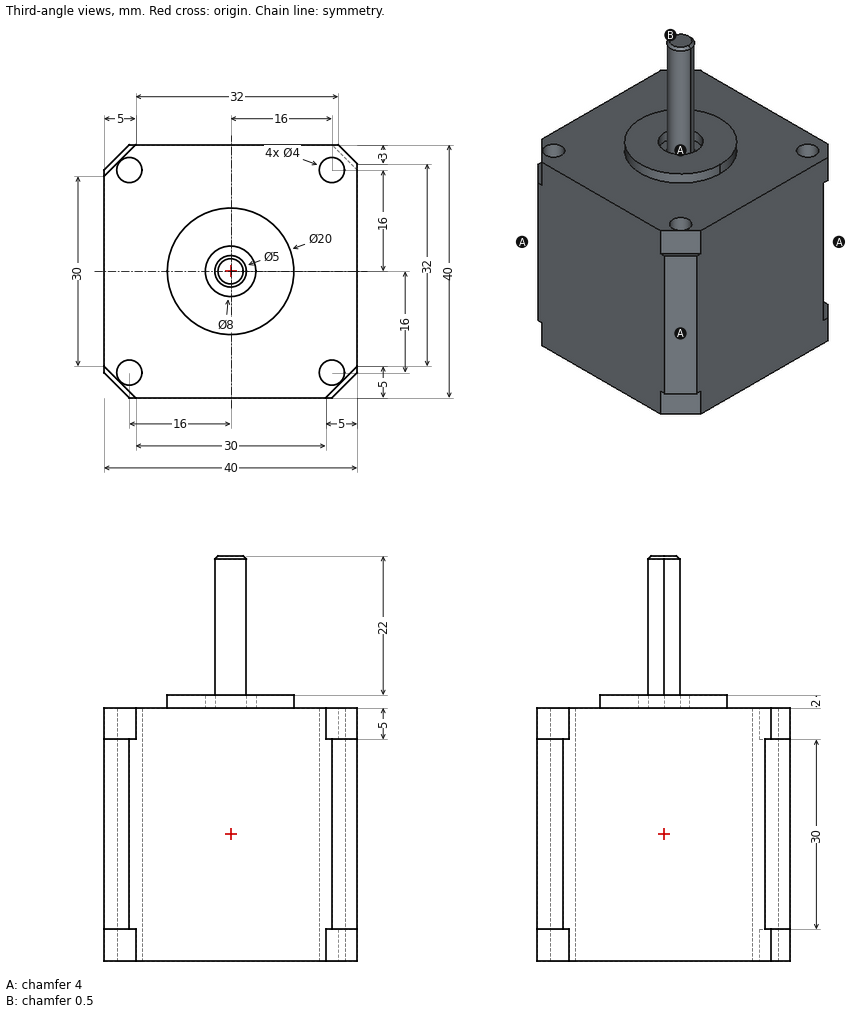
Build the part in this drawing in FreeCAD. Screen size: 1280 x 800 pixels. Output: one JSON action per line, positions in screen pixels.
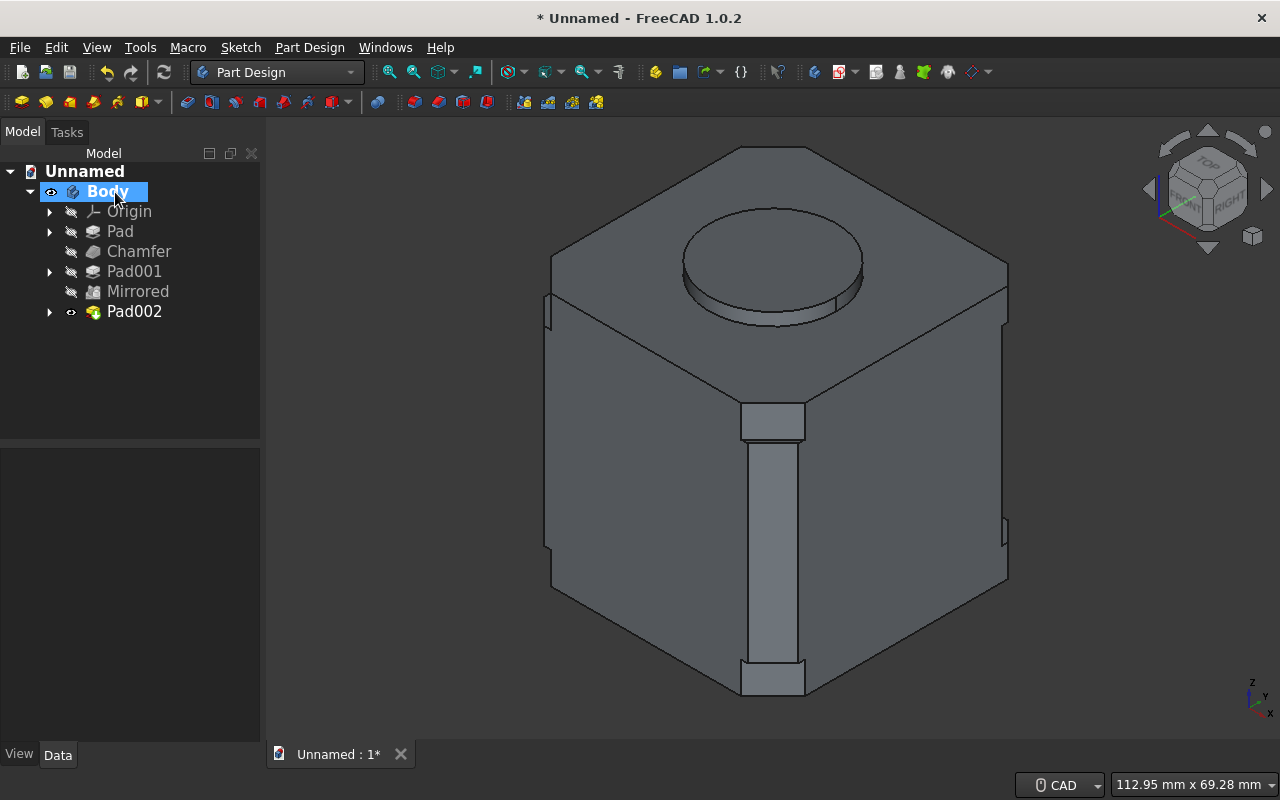
{"action": "left_click", "coordinate": [390, 72]}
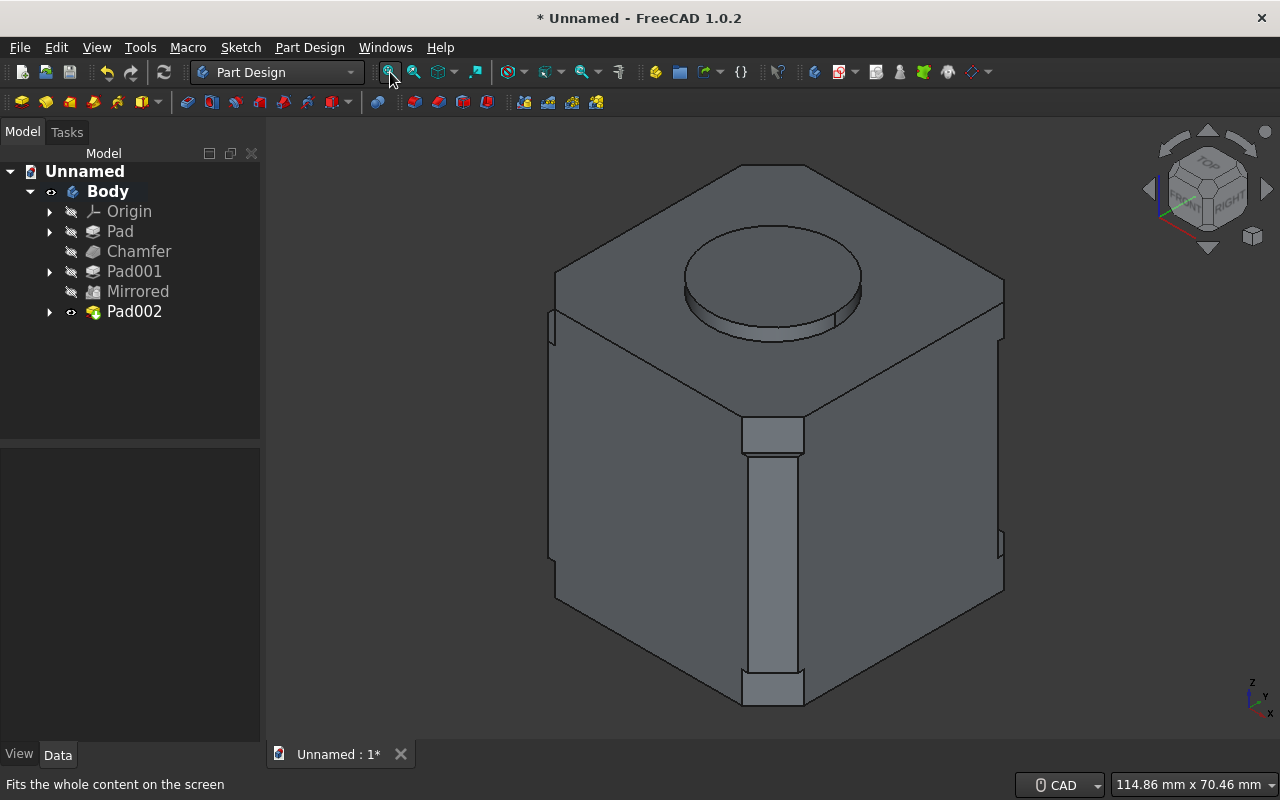
{"action": "left_click", "coordinate": [773, 276]}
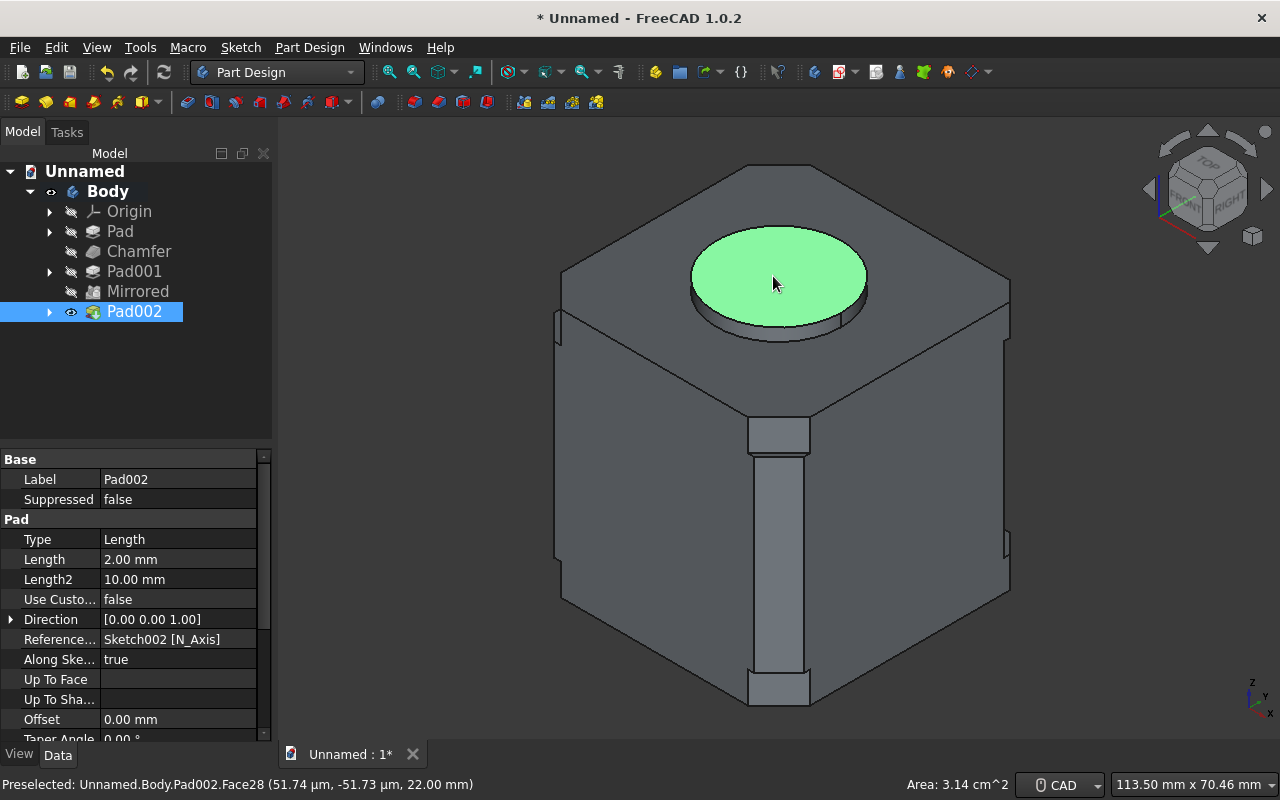
{"action": "left_click", "coordinate": [840, 72]}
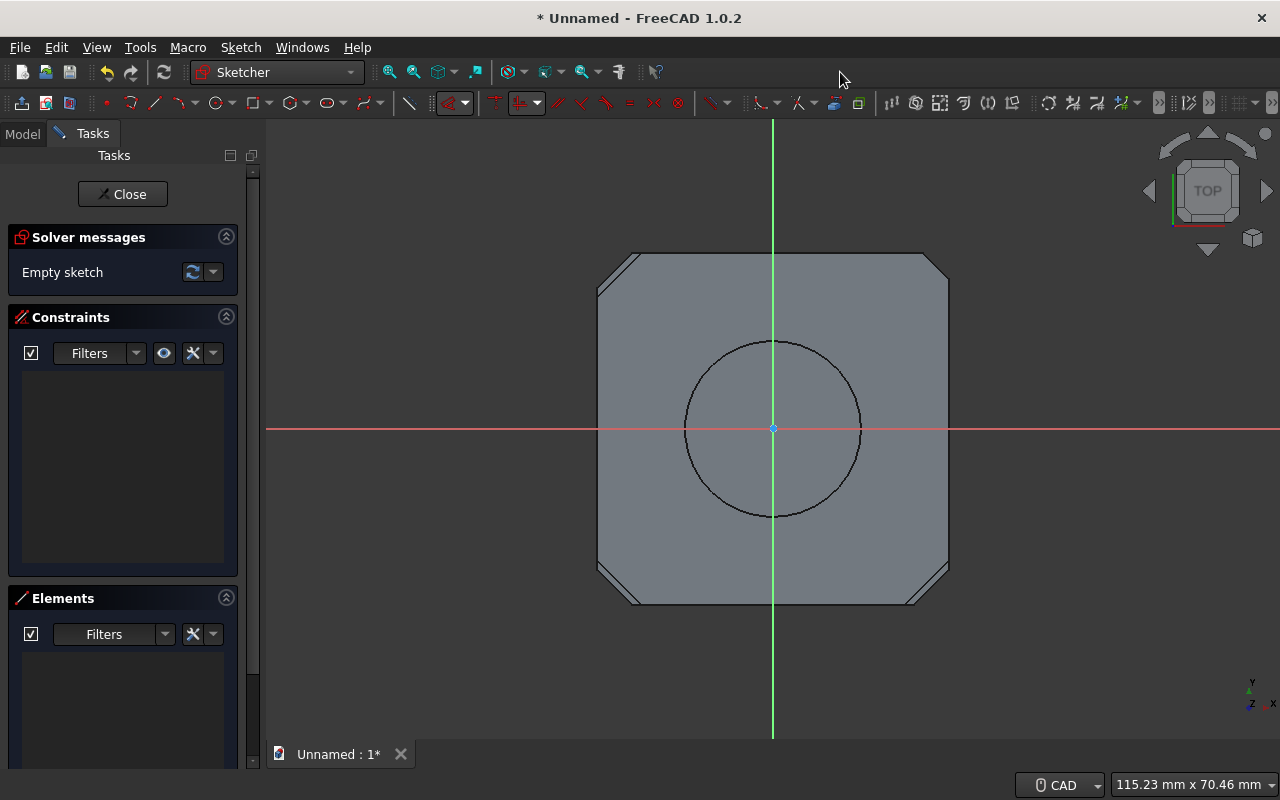
{"action": "scroll", "coordinate": [782, 429], "scroll_direction": "up", "scroll_amount": 11}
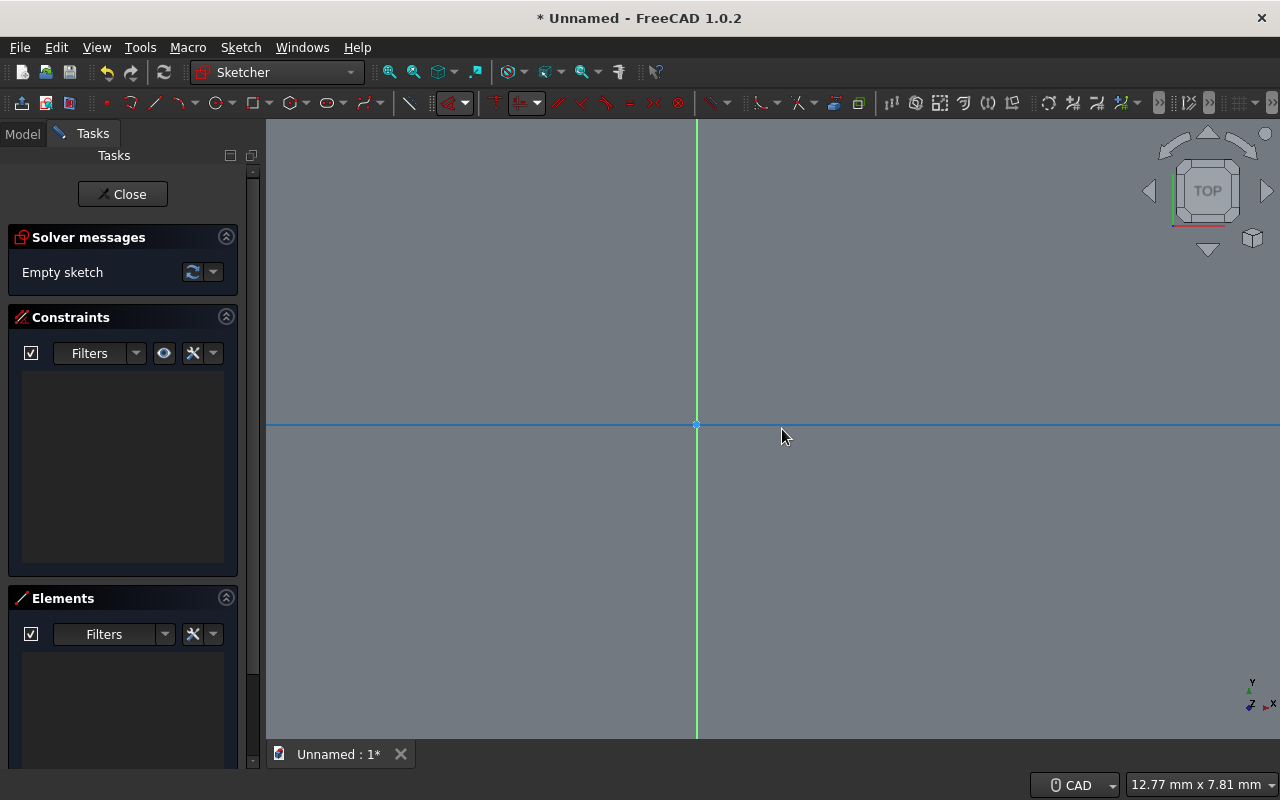
{"action": "key", "text": "g c"}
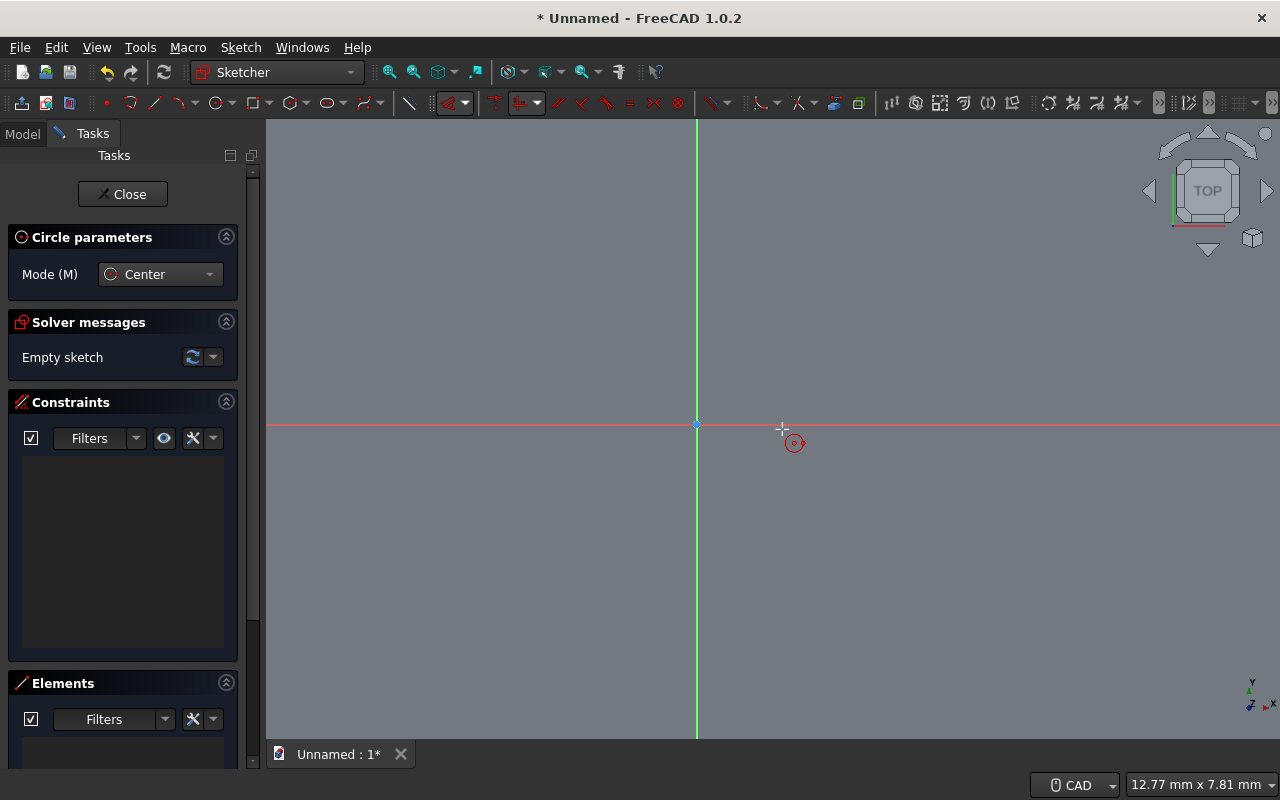
{"action": "left_click", "coordinate": [697, 425]}
{"action": "mouse_move", "coordinate": [837, 285]}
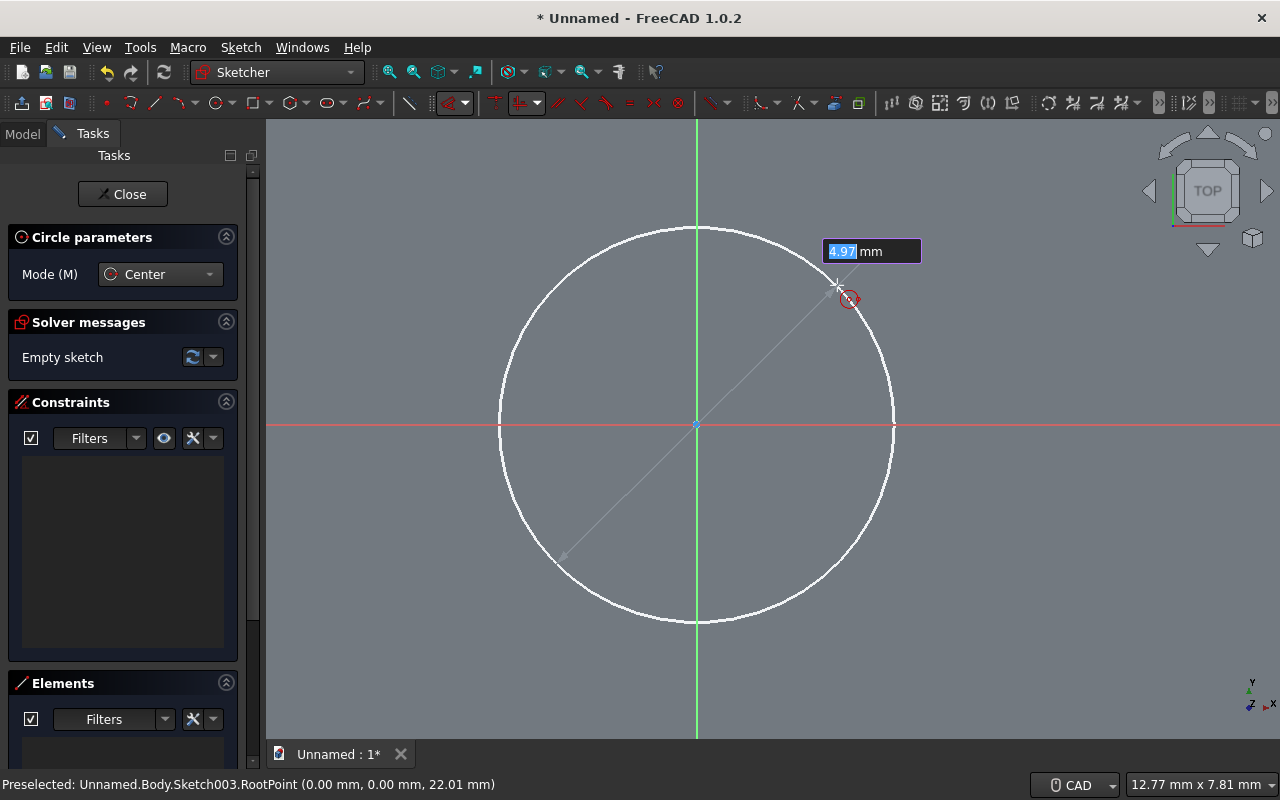
{"action": "type", "text": "5"}
{"action": "key", "text": "Return"}
{"action": "key", "text": "Escape"}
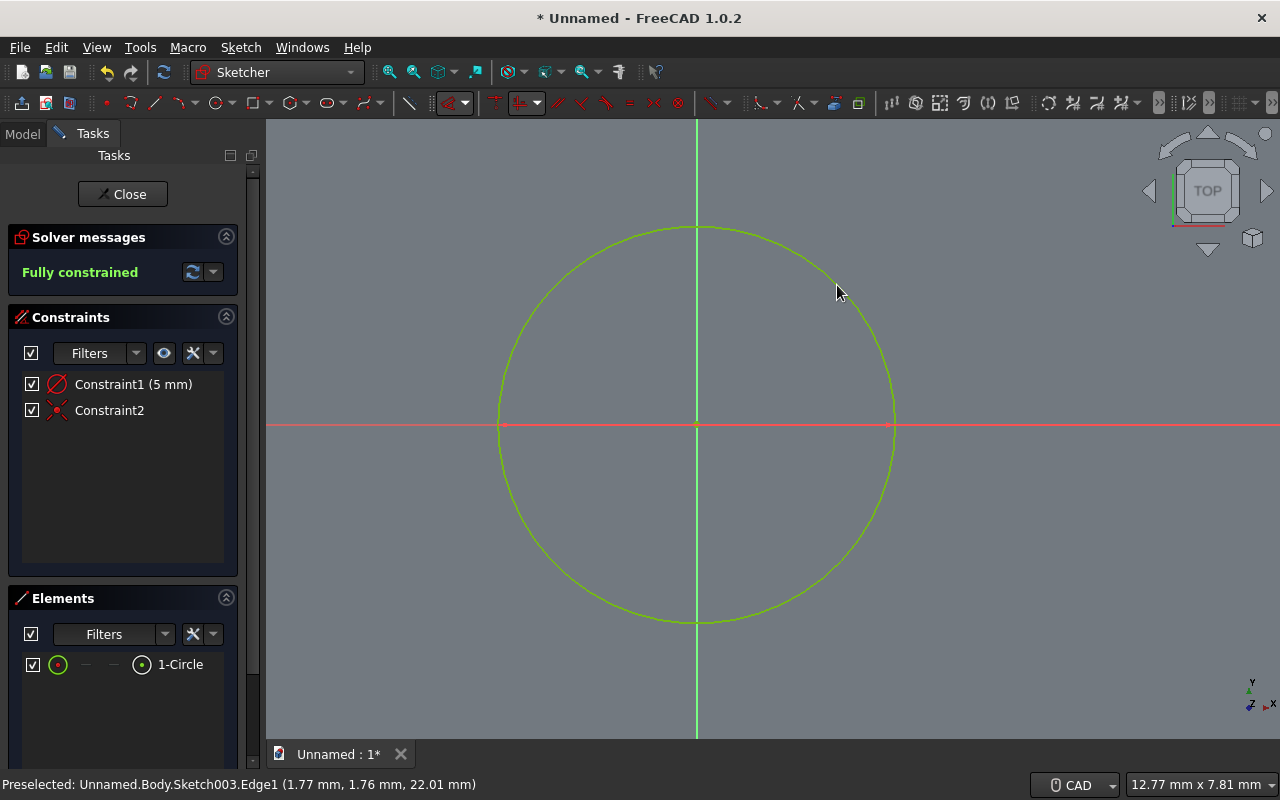
{"action": "left_click", "coordinate": [123, 194]}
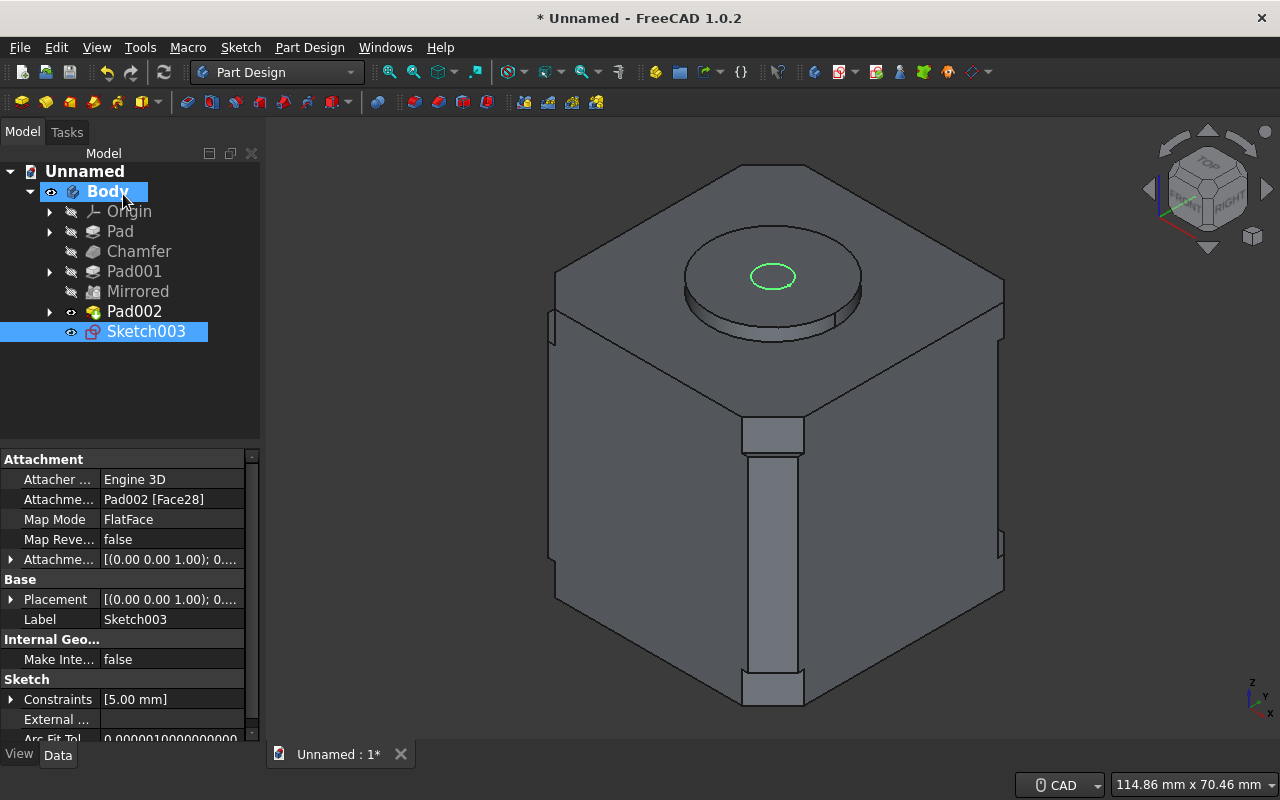
{"action": "left_click", "coordinate": [22, 102]}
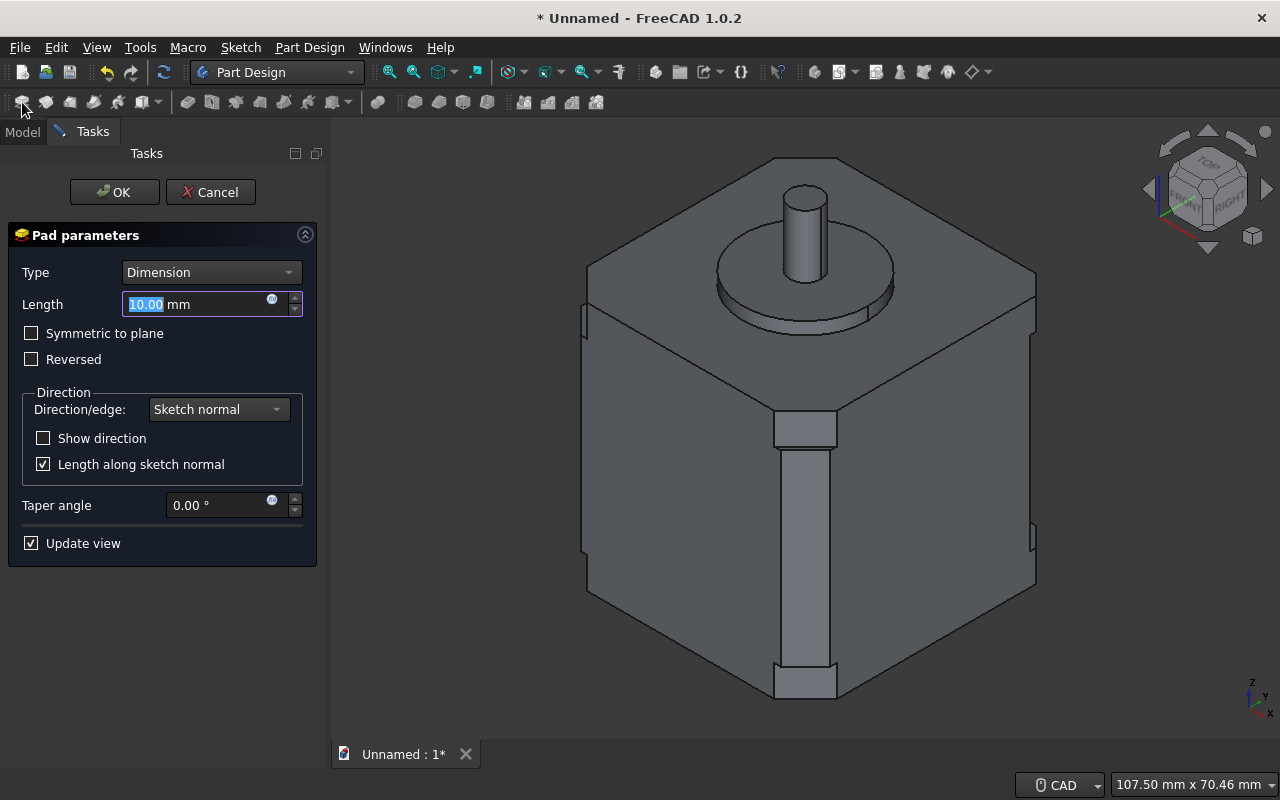
{"action": "type", "text": "22"}
{"action": "key", "text": "Tab"}